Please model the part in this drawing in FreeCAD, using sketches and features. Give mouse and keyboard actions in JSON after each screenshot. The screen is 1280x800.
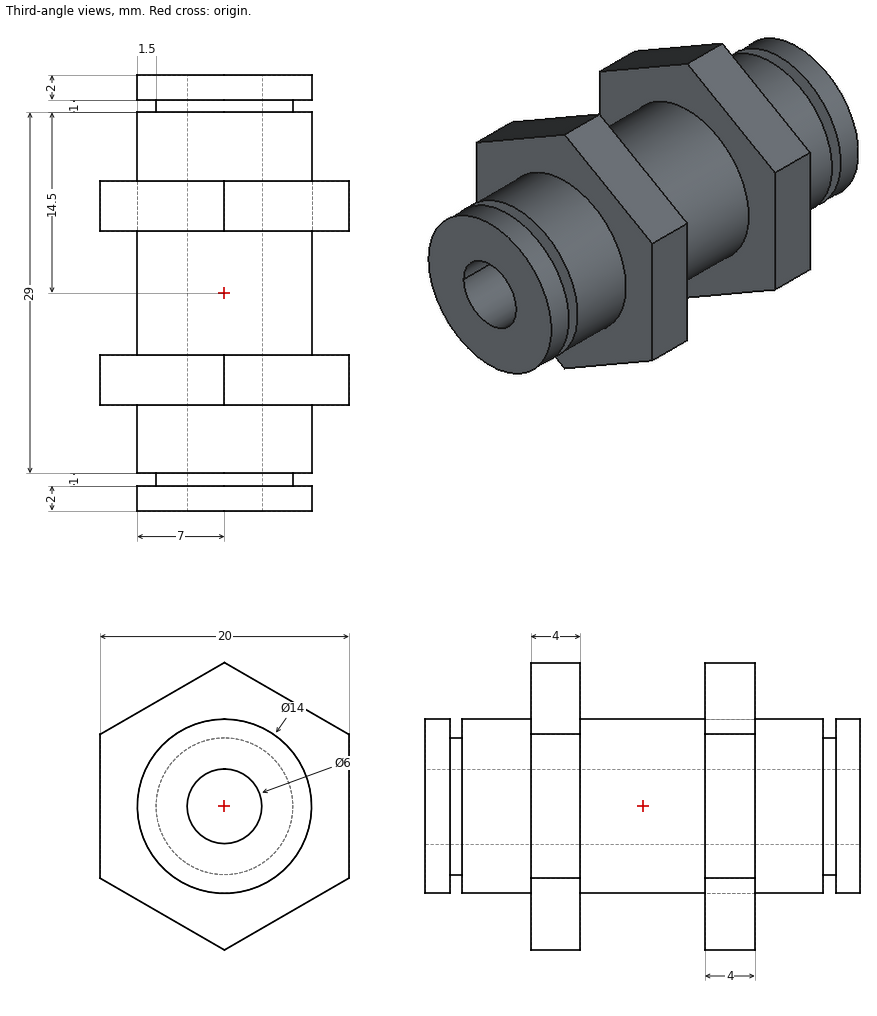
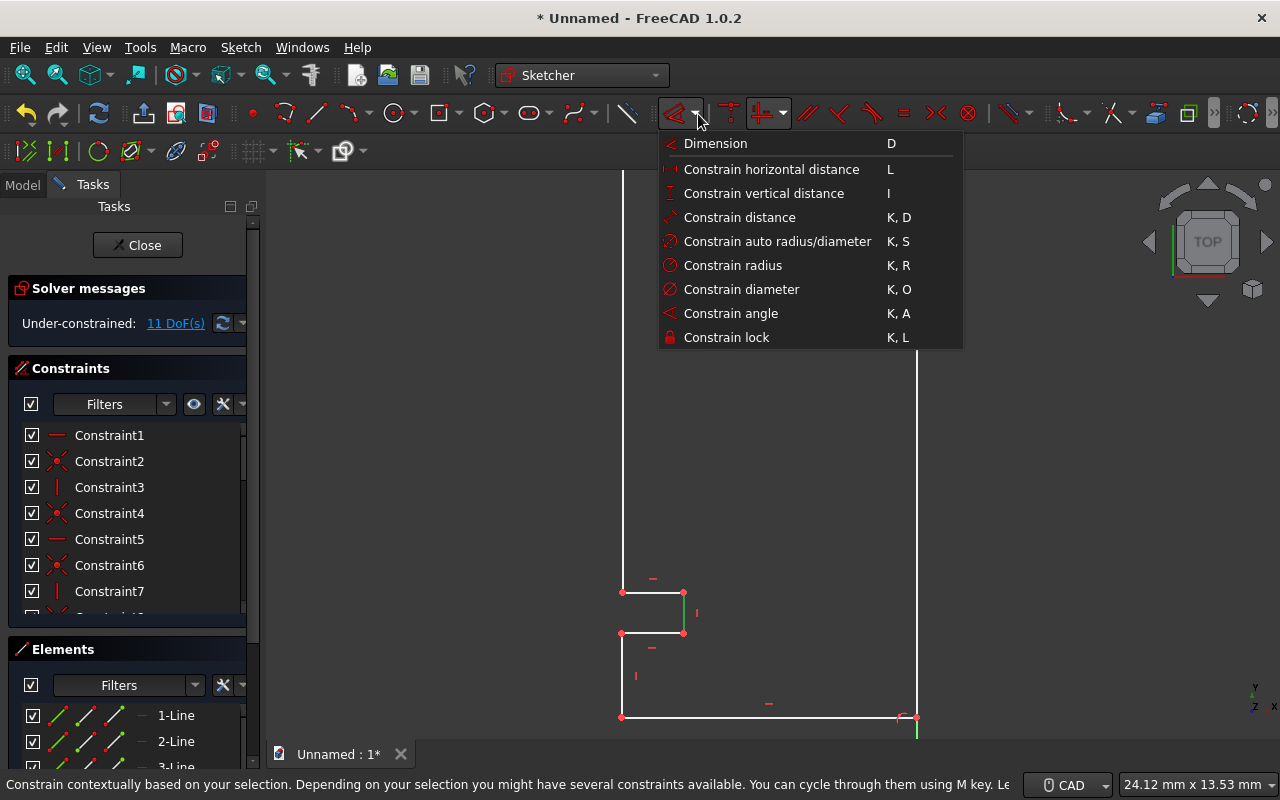
{"action": "left_click", "coordinate": [811, 193]}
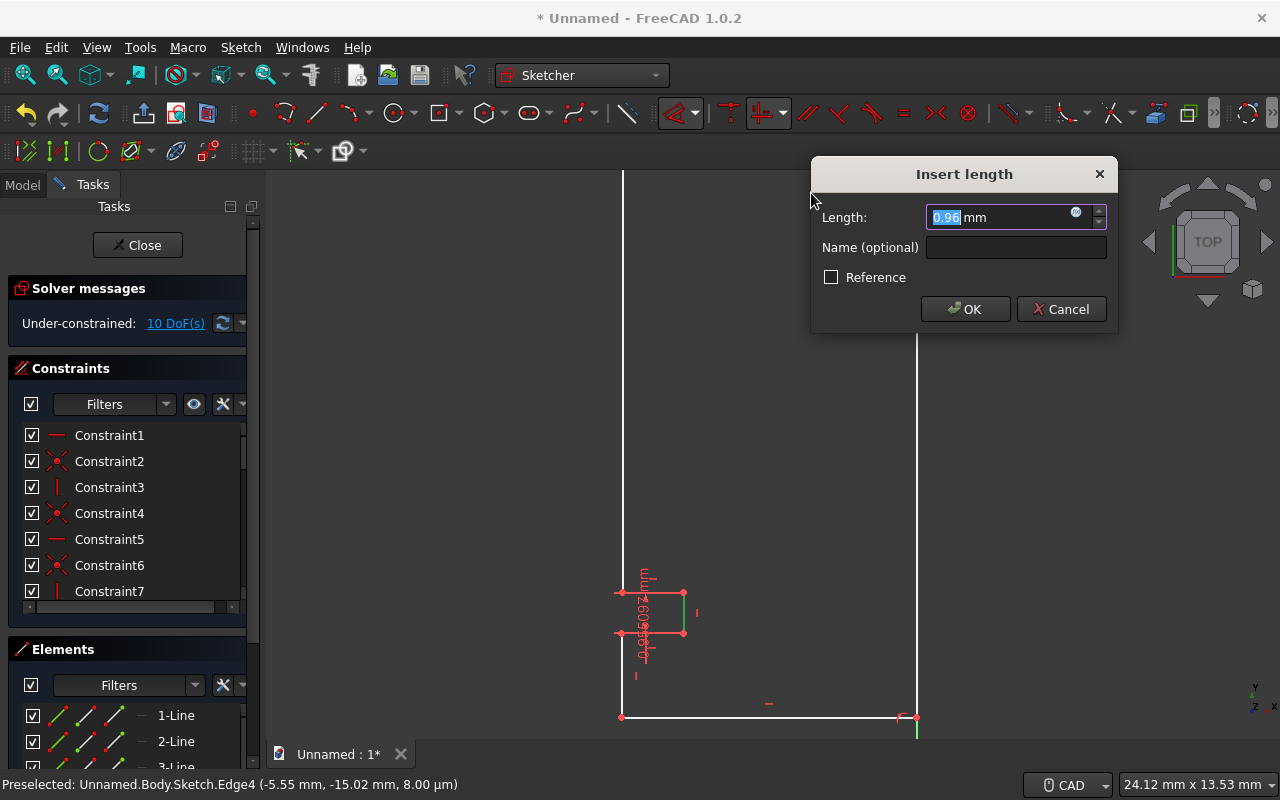
{"action": "type", "text": "1"}
{"action": "key", "text": "Return"}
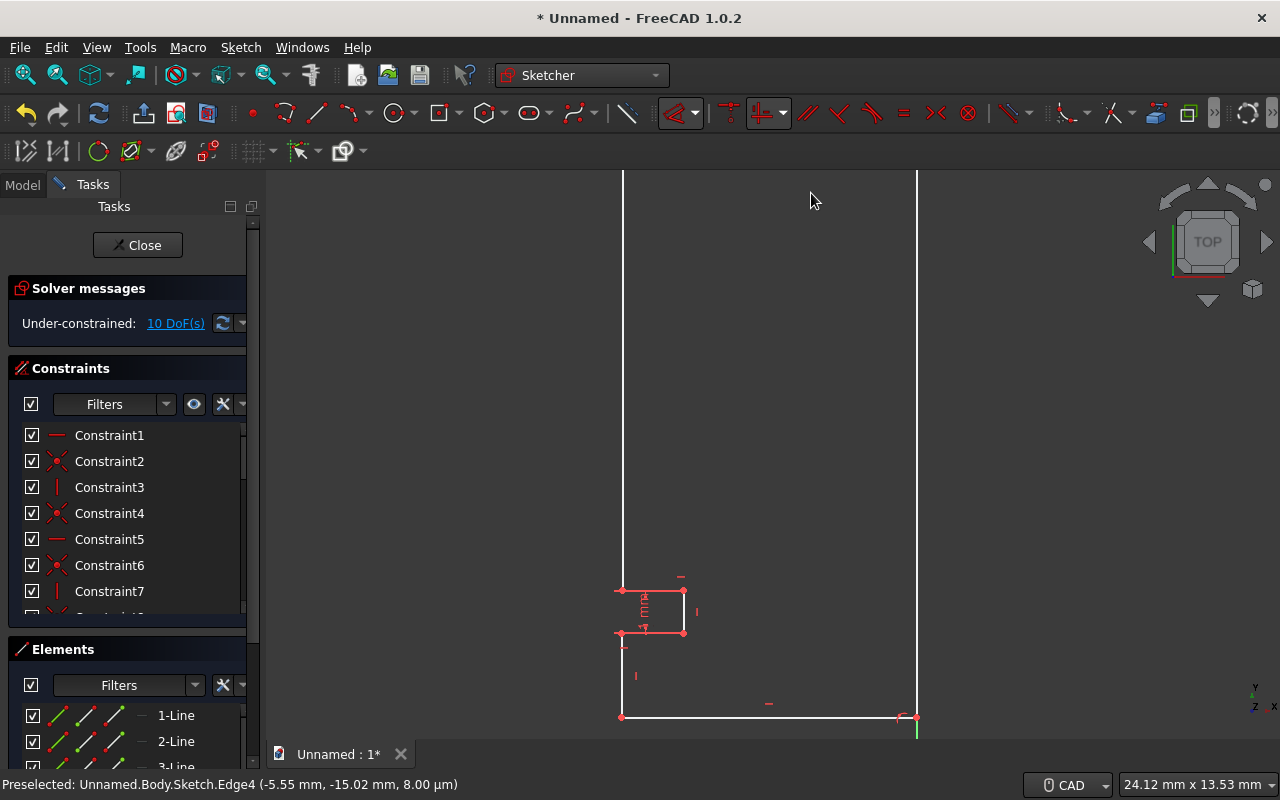
{"action": "left_click", "coordinate": [622, 658]}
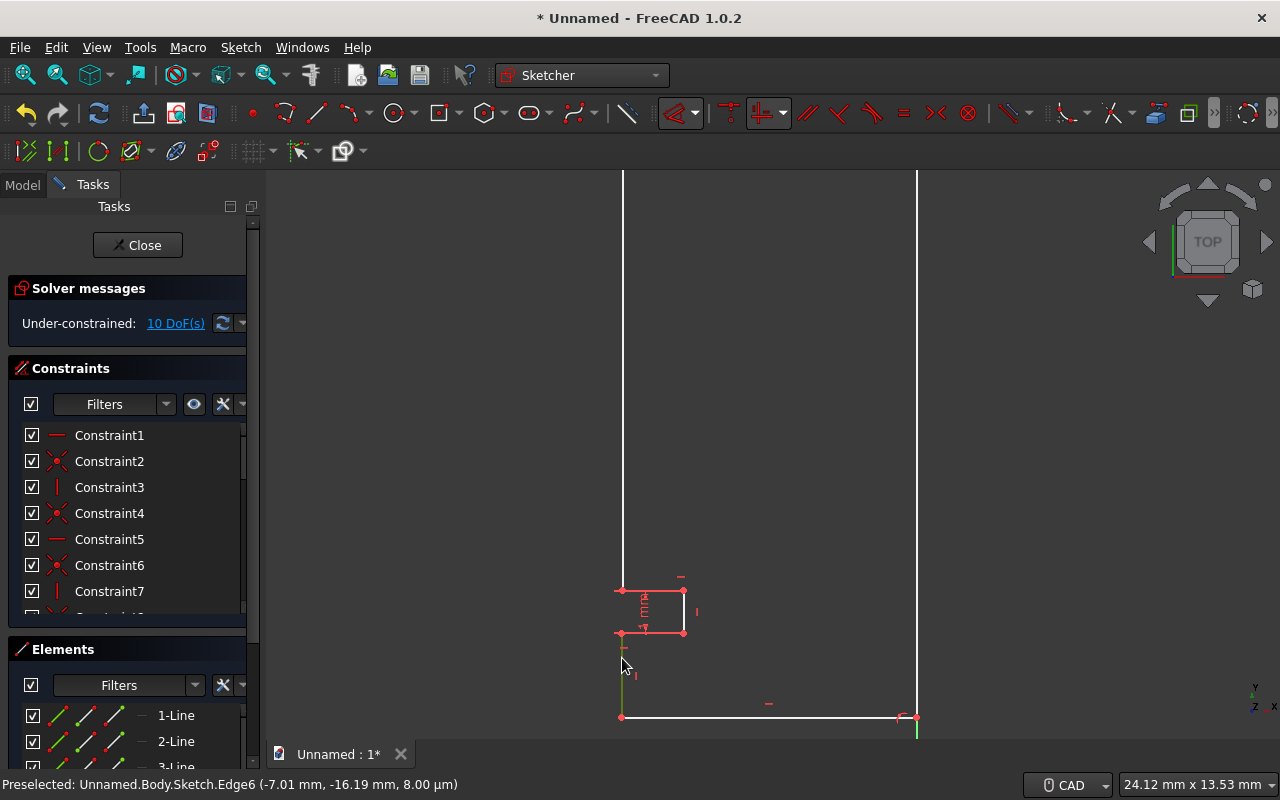
{"action": "left_click", "coordinate": [698, 114]}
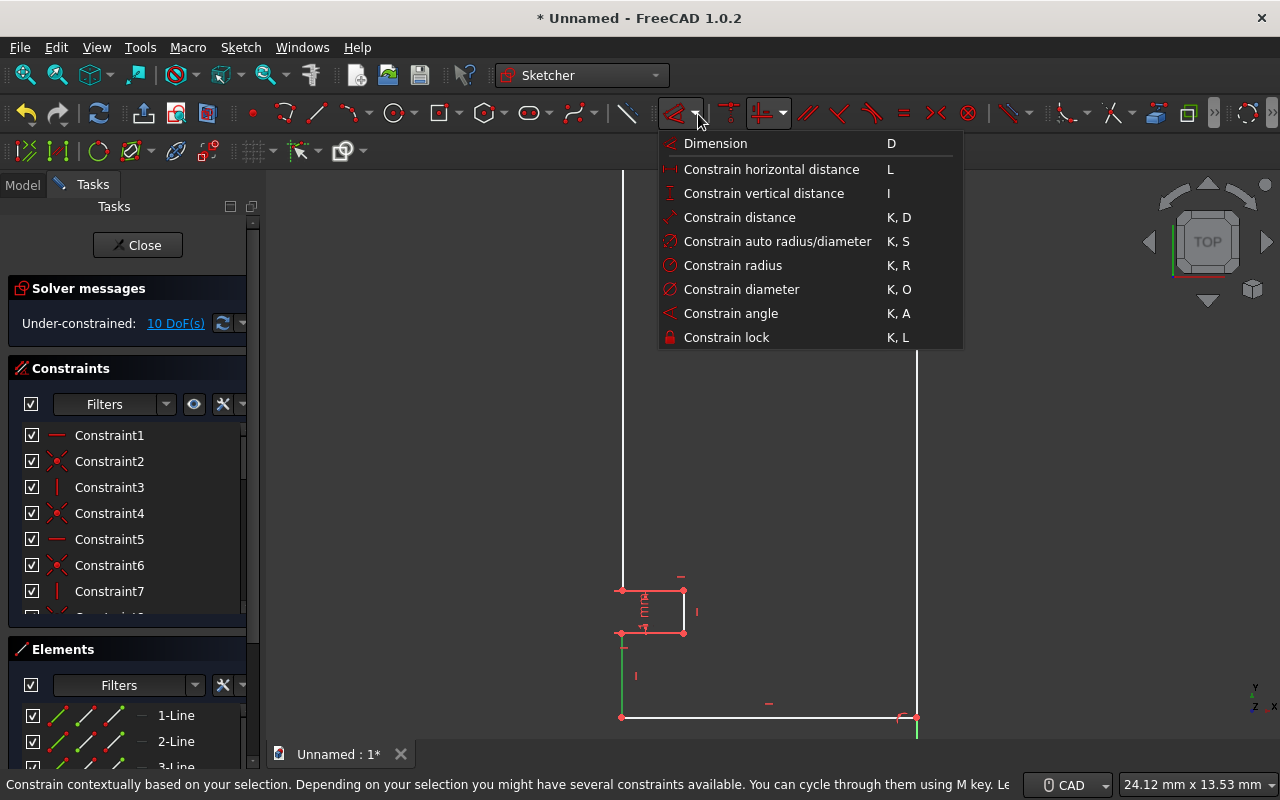
{"action": "left_click", "coordinate": [811, 193]}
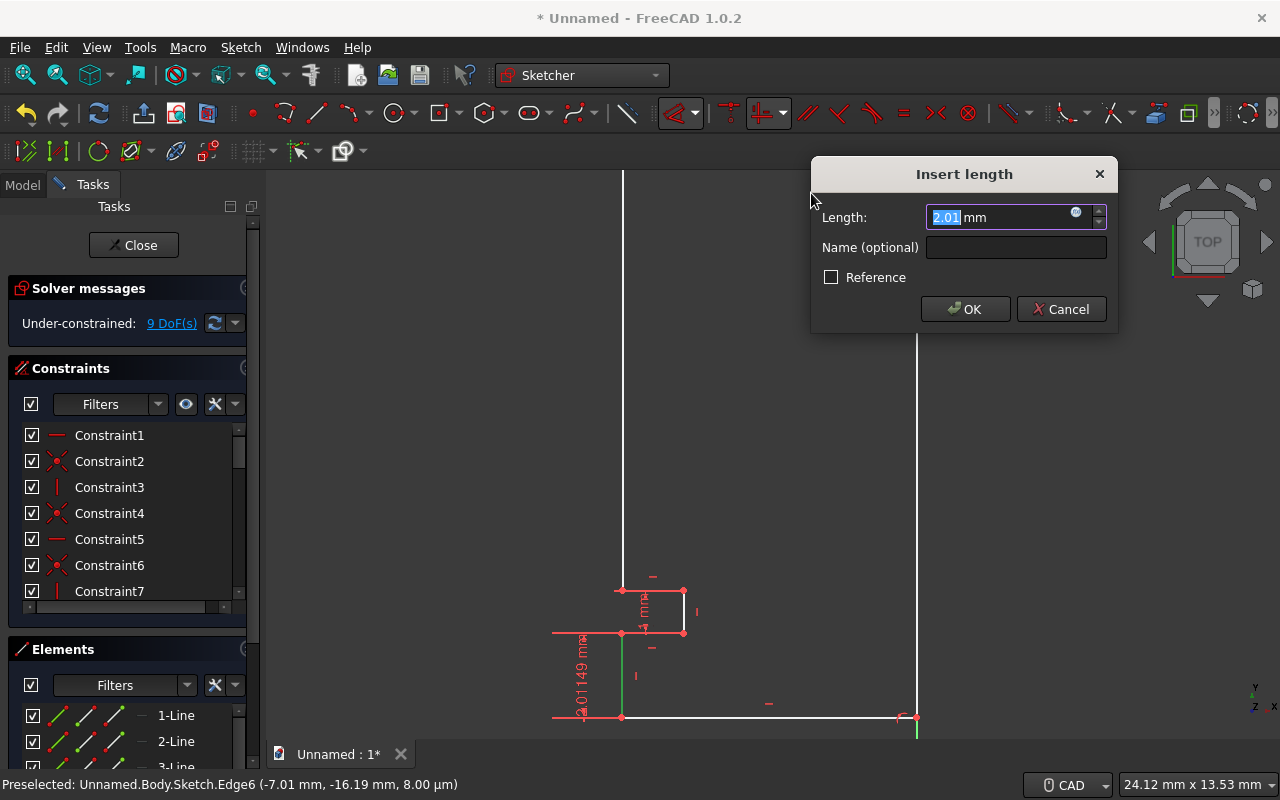
{"action": "type", "text": "2"}
{"action": "key", "text": "Return"}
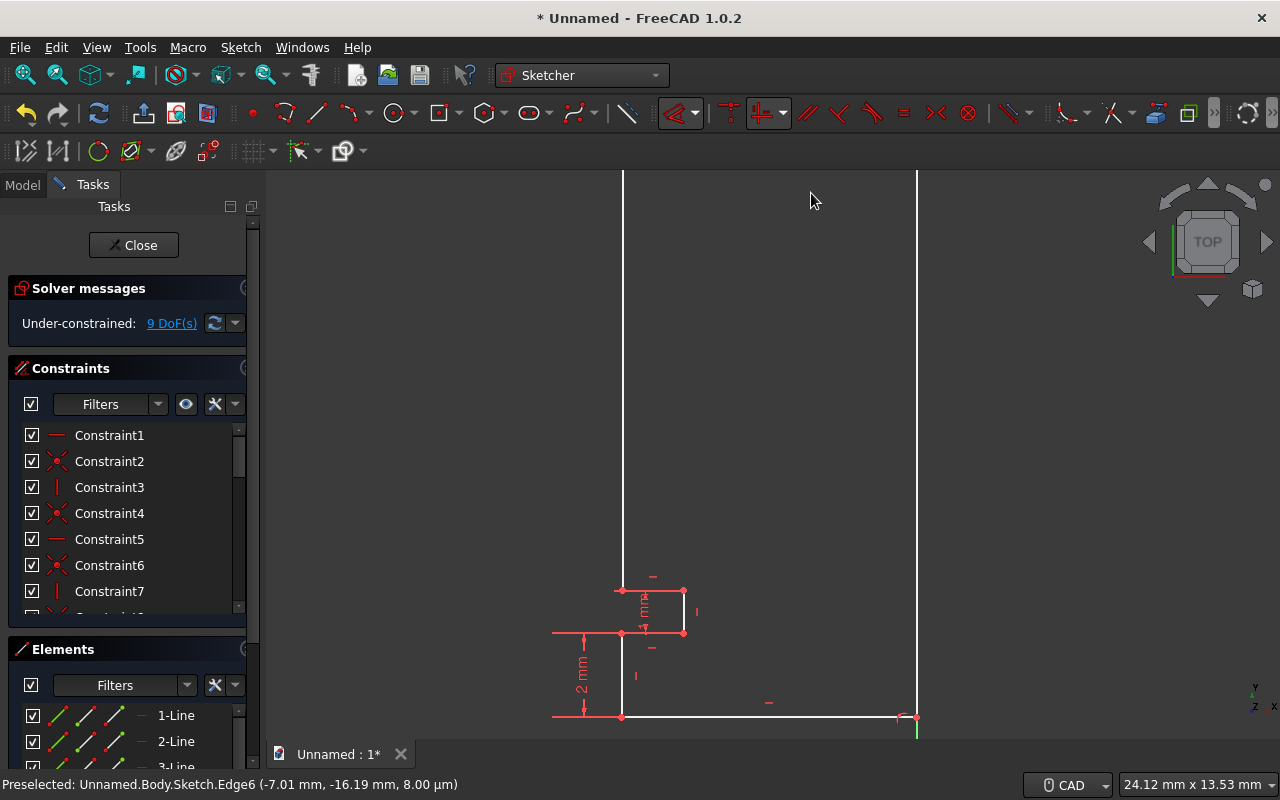
{"action": "scroll", "coordinate": [683, 610], "scroll_direction": "down", "scroll_amount": 7}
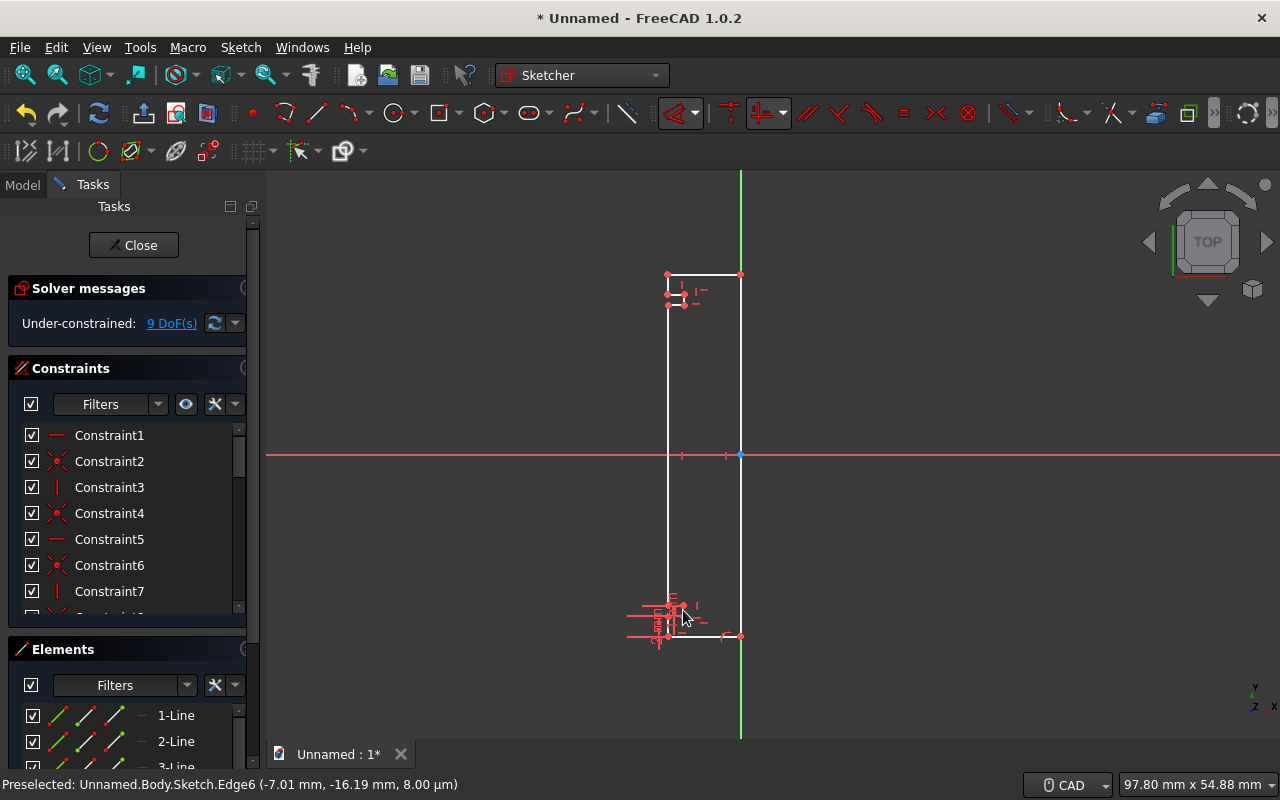
{"action": "left_click", "coordinate": [690, 637]}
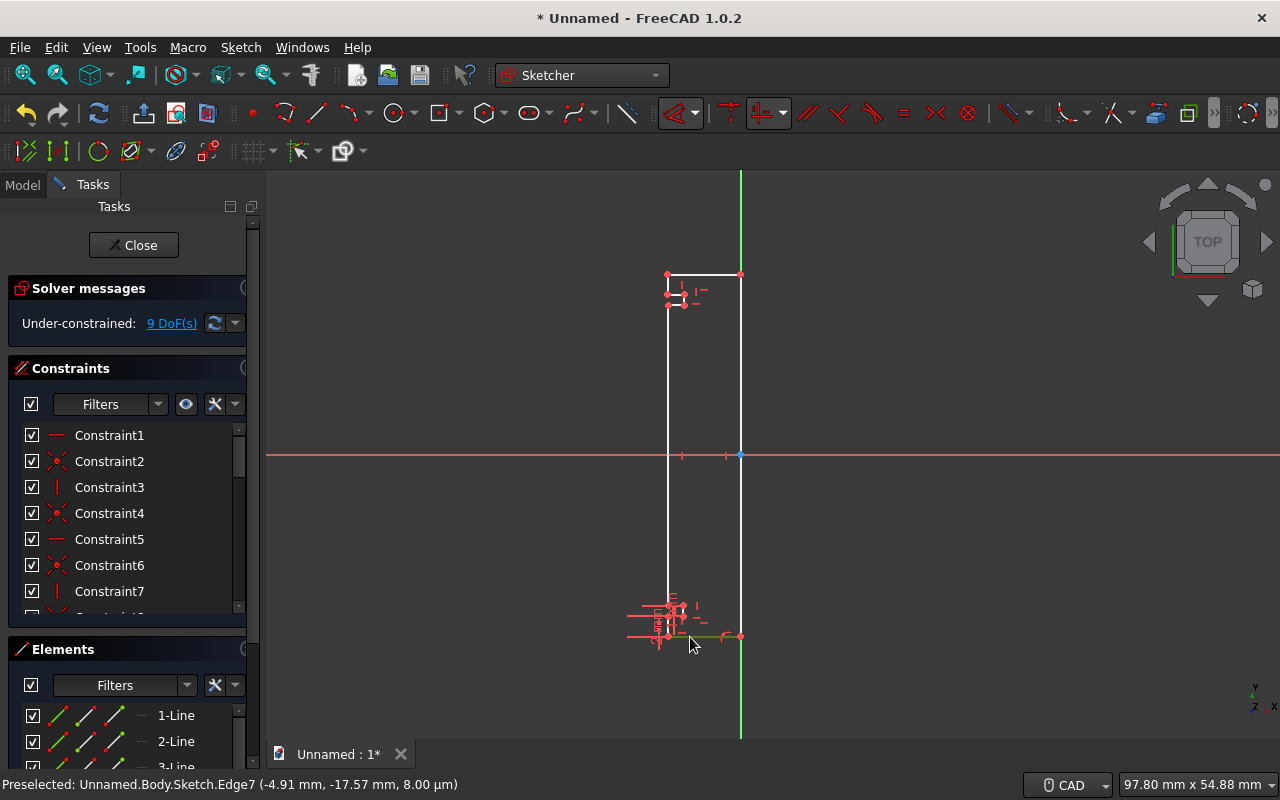
{"action": "left_click", "coordinate": [698, 114]}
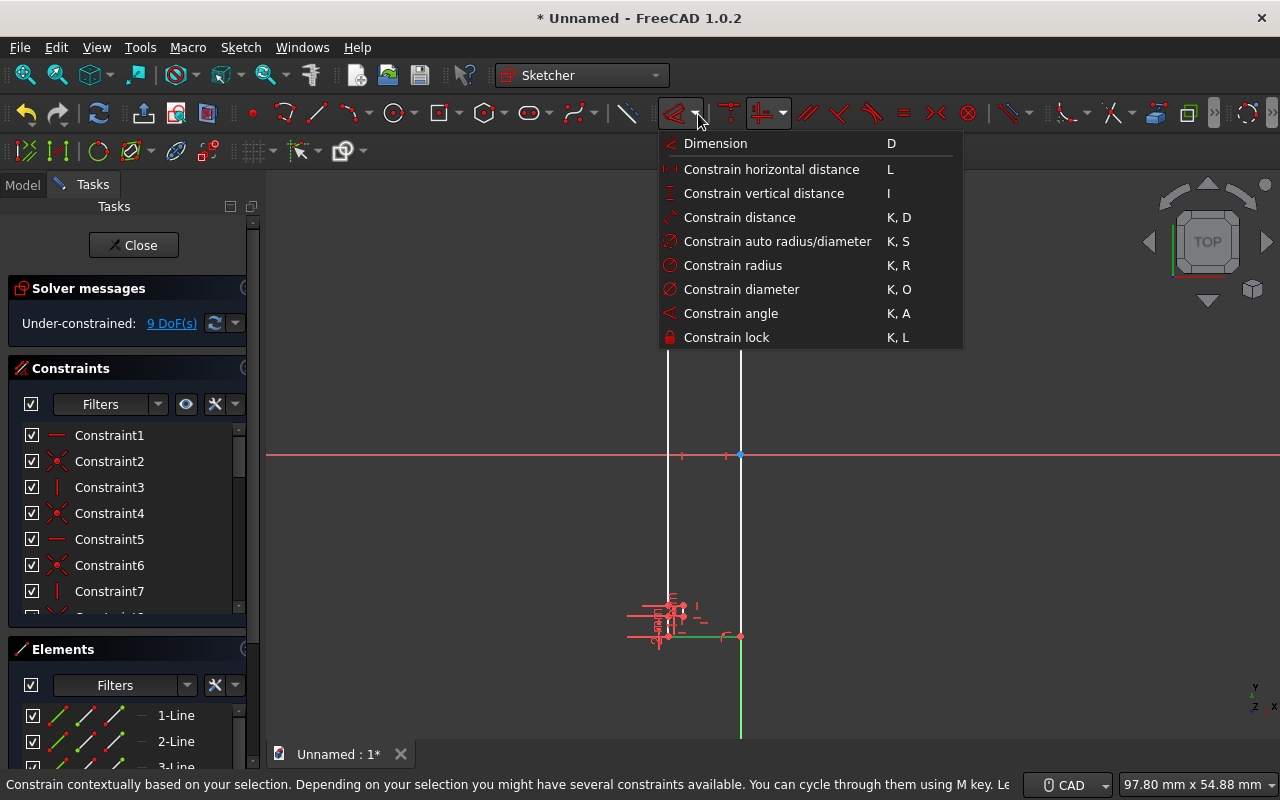
{"action": "left_click", "coordinate": [811, 169]}